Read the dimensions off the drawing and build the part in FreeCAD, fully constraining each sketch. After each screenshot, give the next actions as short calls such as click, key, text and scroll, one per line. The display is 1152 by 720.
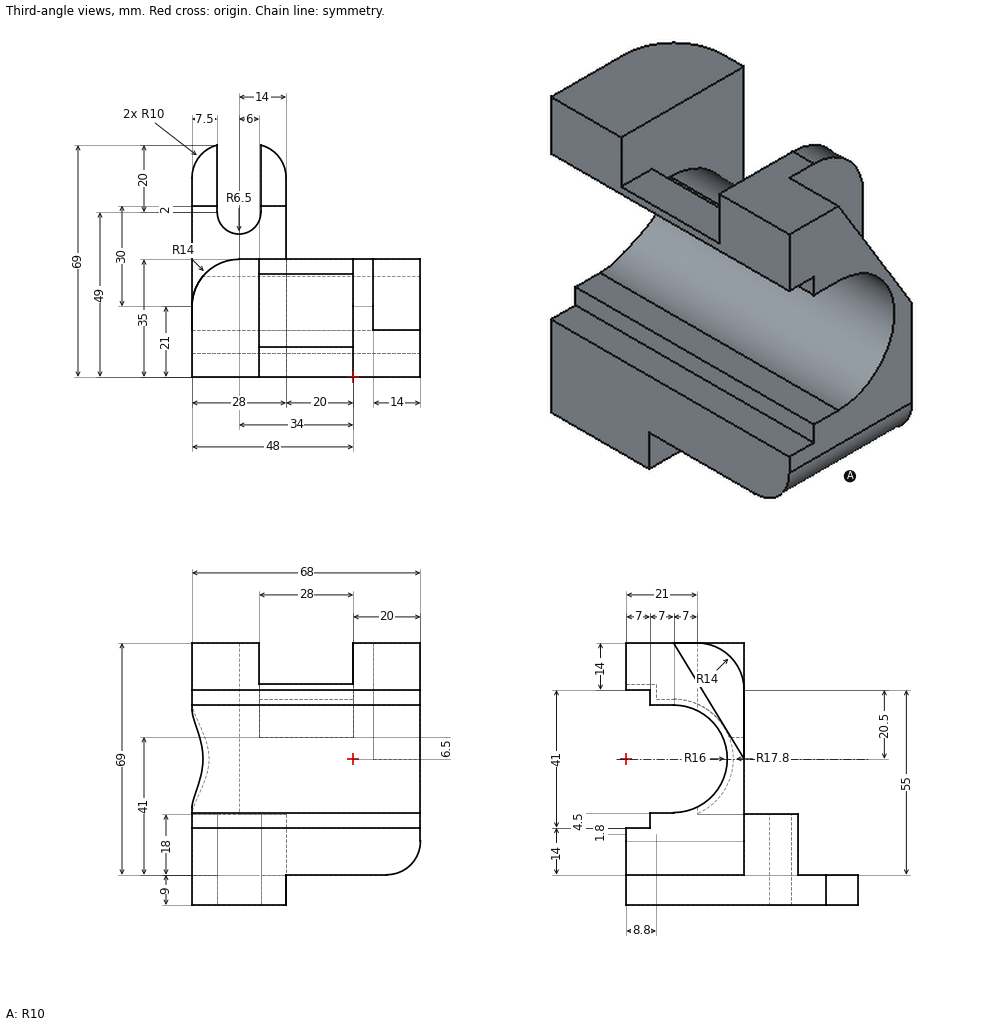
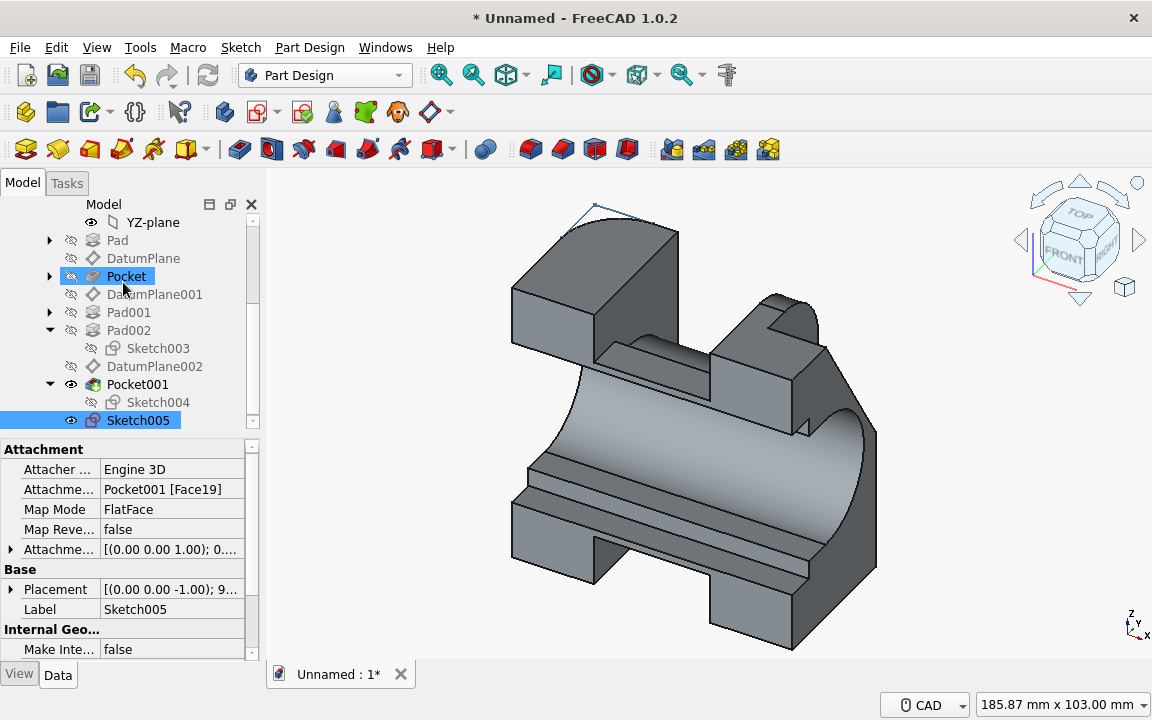
click(240, 150)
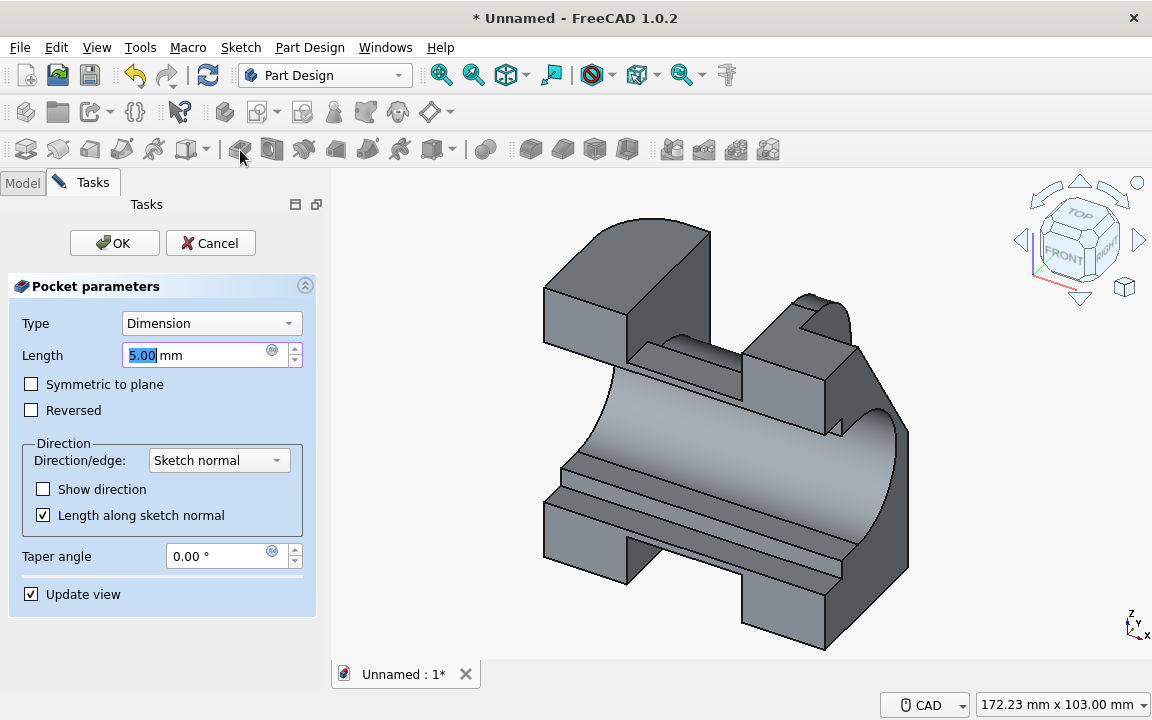
text(69)
key(Tab)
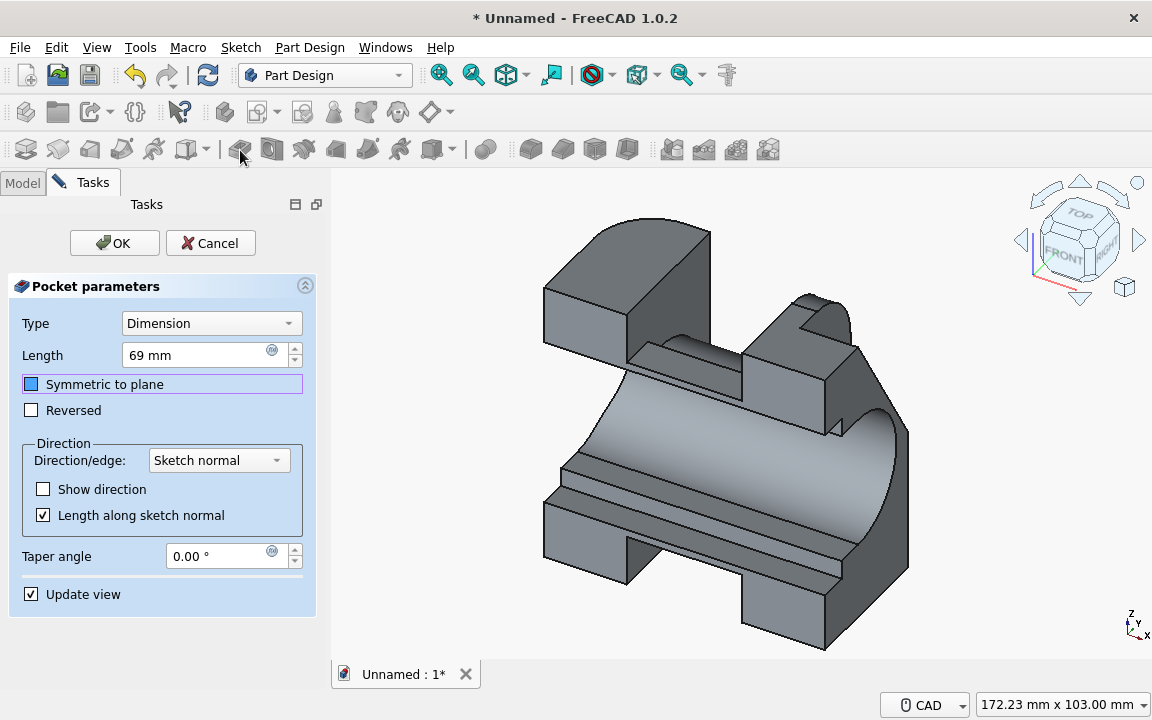
click(115, 243)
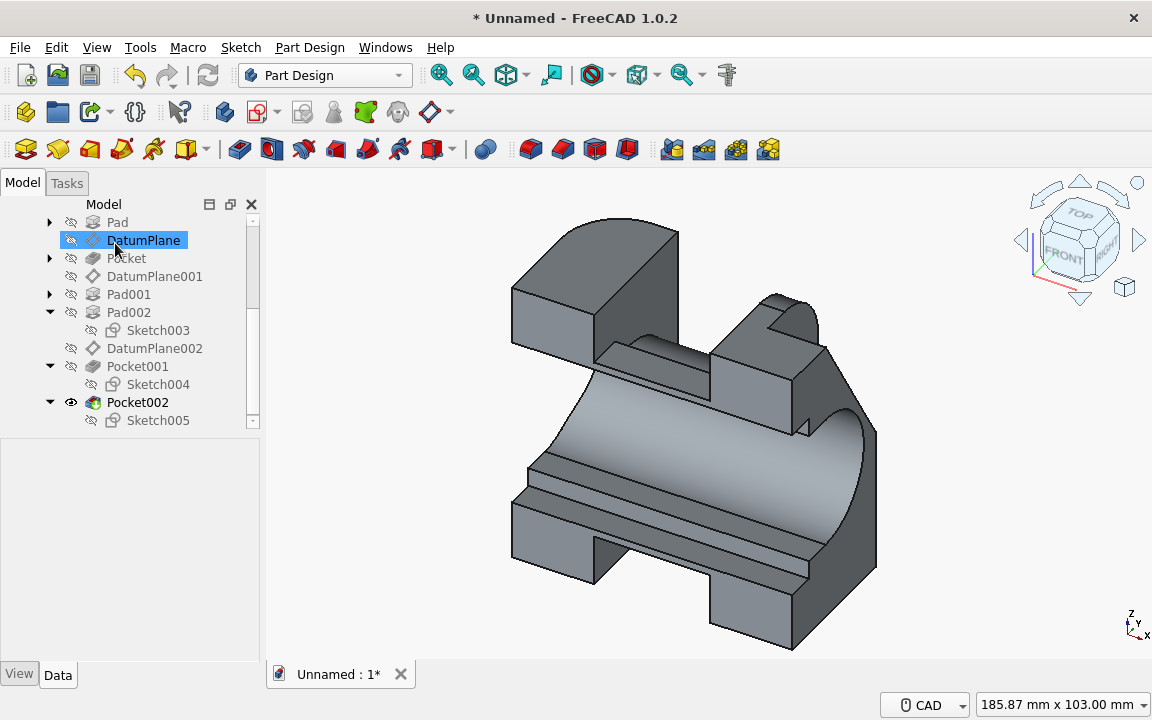
key(5)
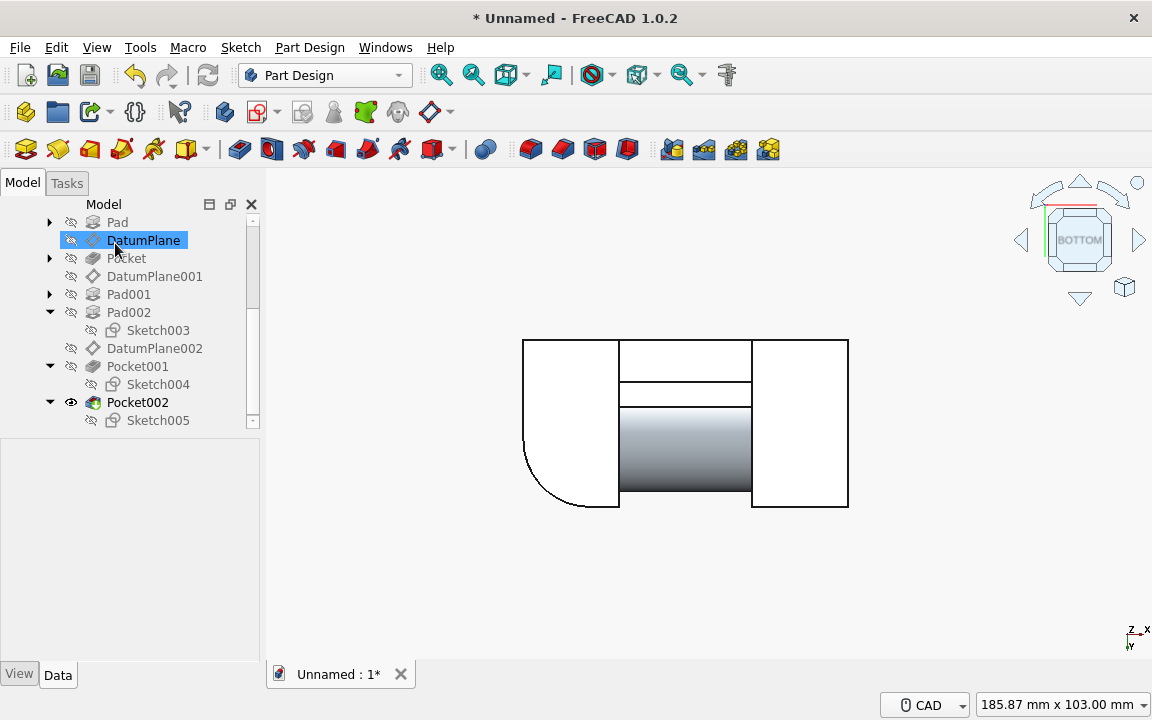
key(v)
key(f)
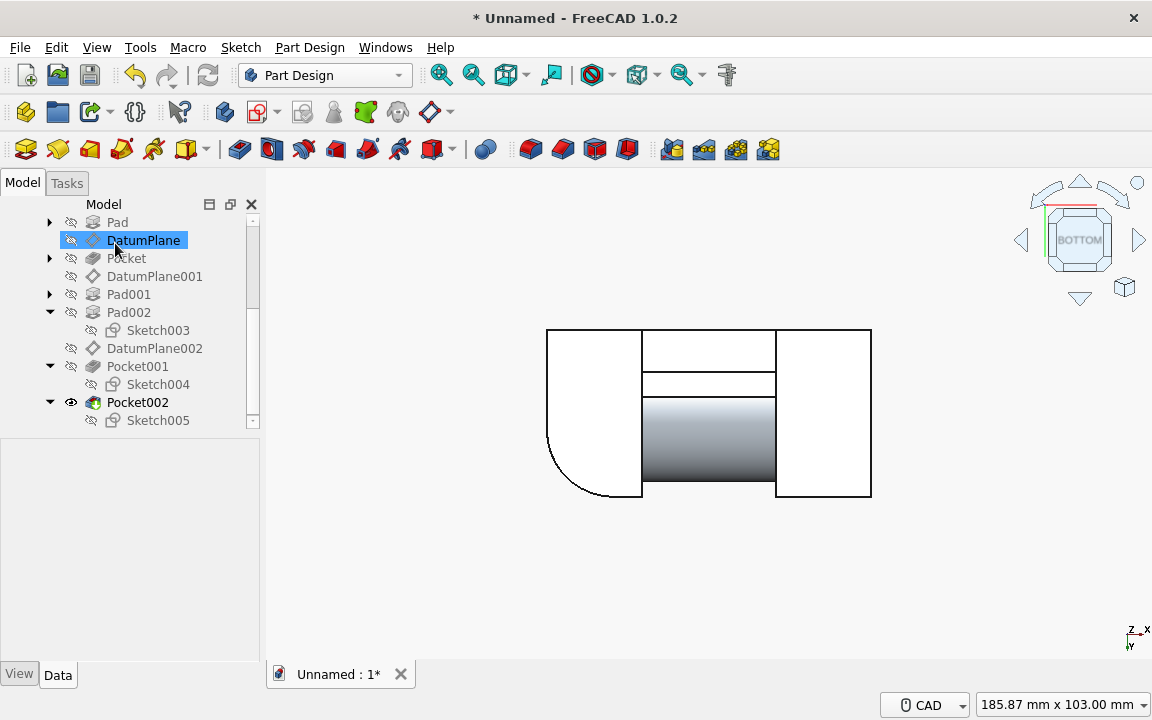
click(823, 436)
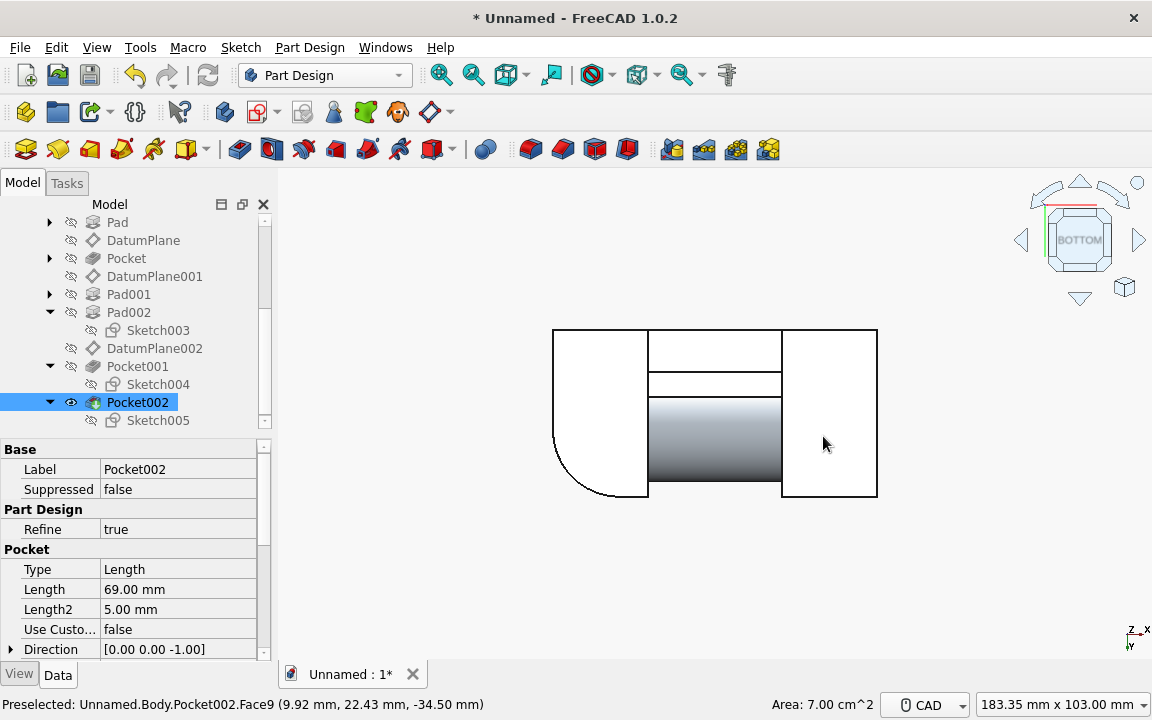
click(258, 112)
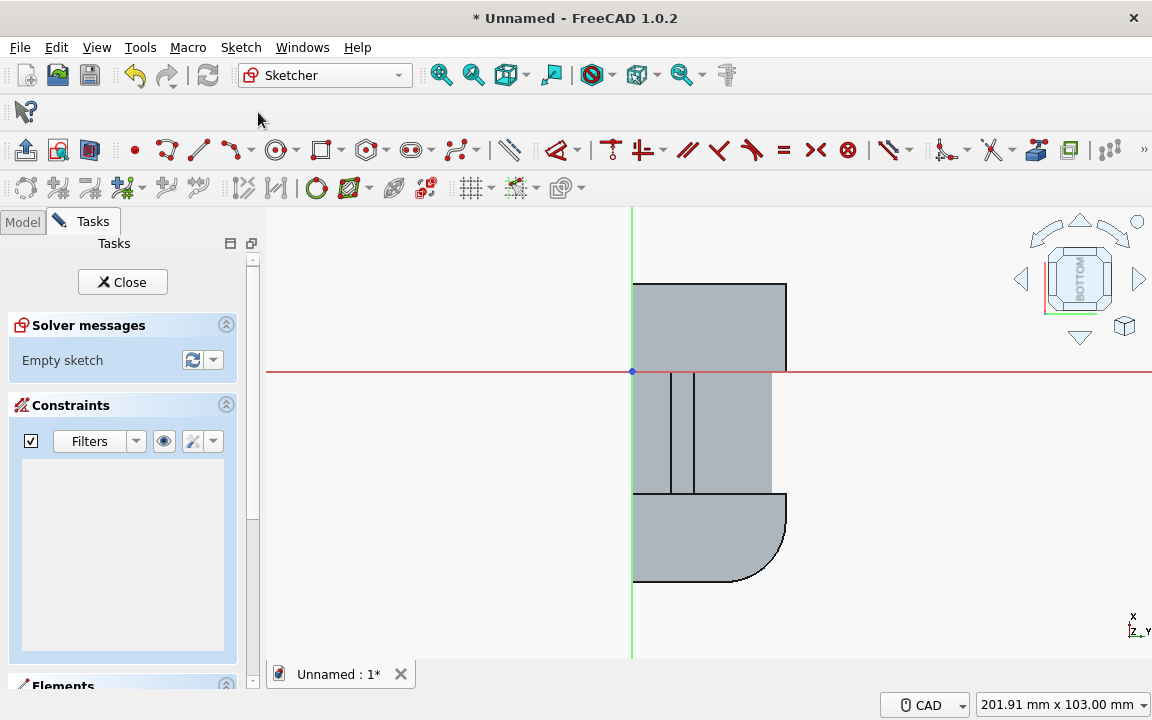
click(200, 150)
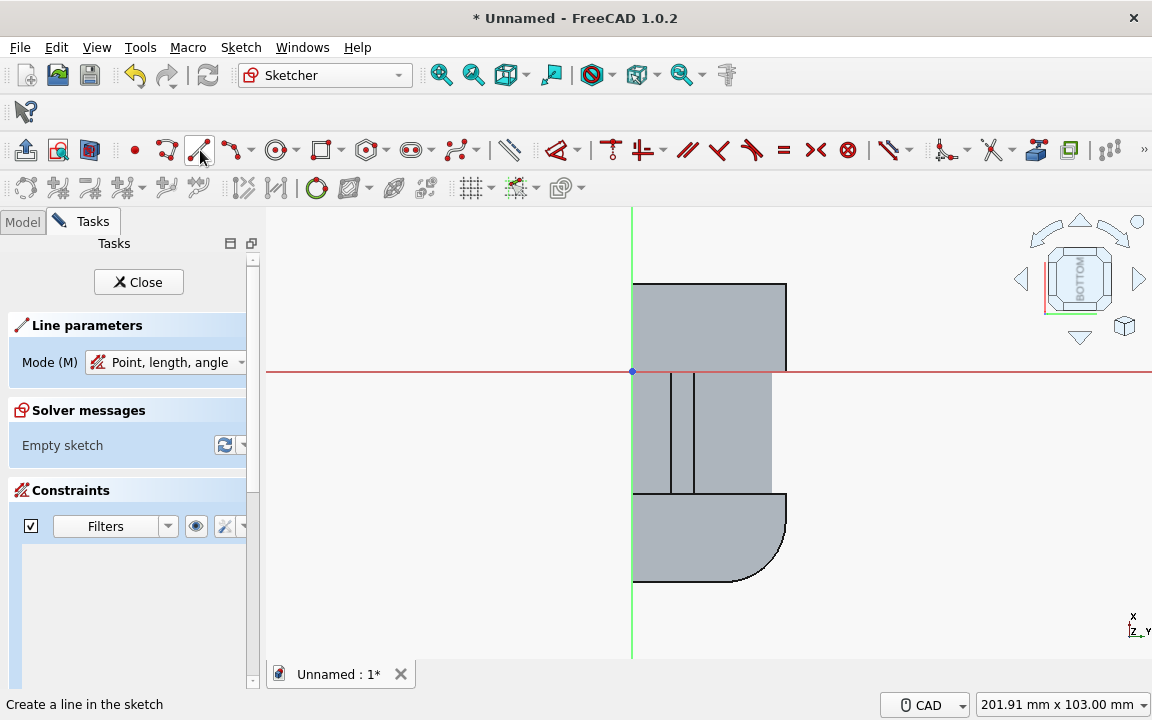
click(935, 549)
click(847, 549)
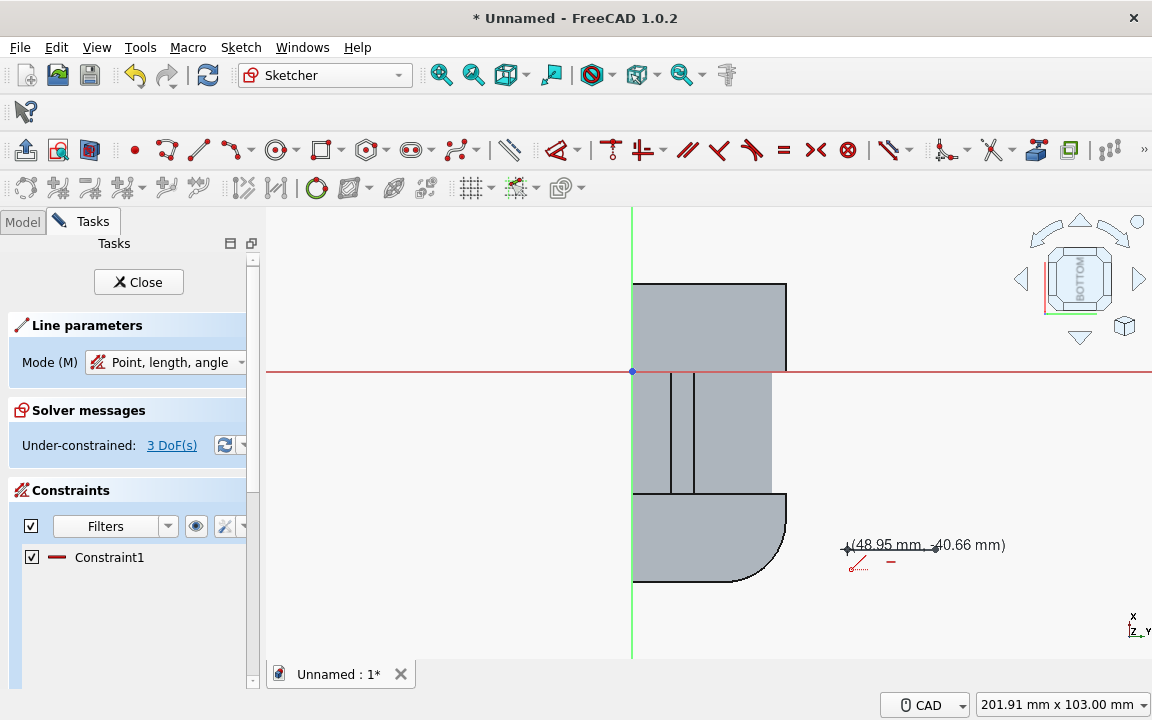
click(847, 492)
click(935, 492)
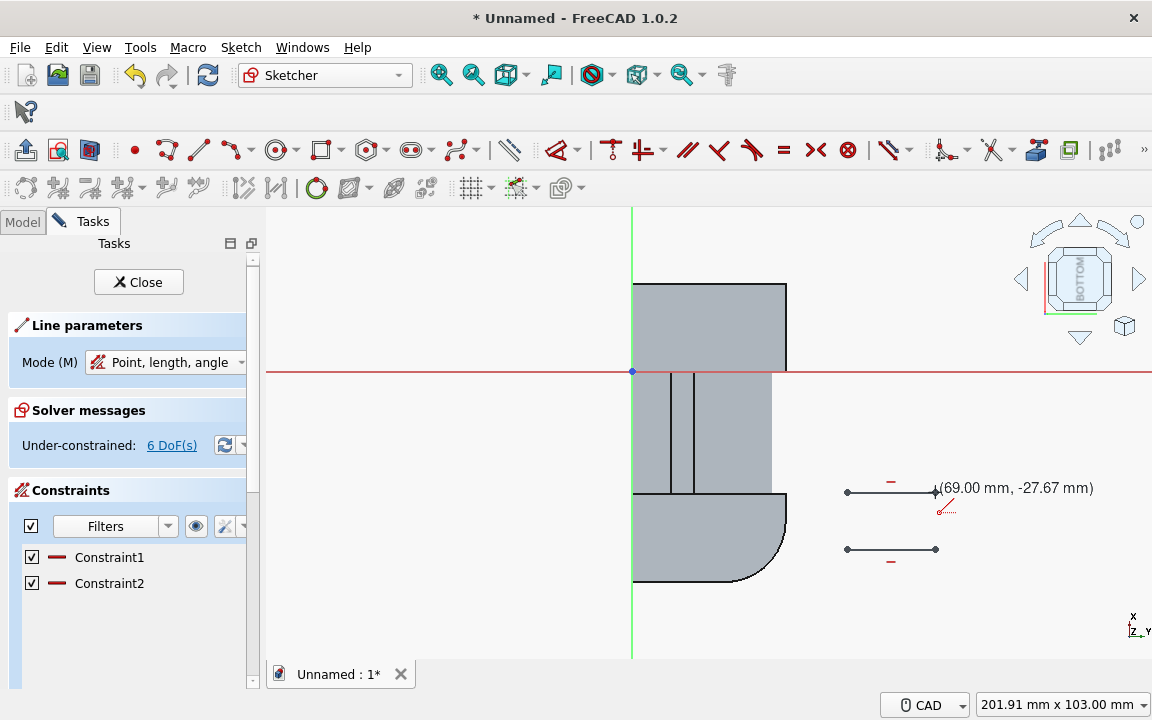
click(168, 150)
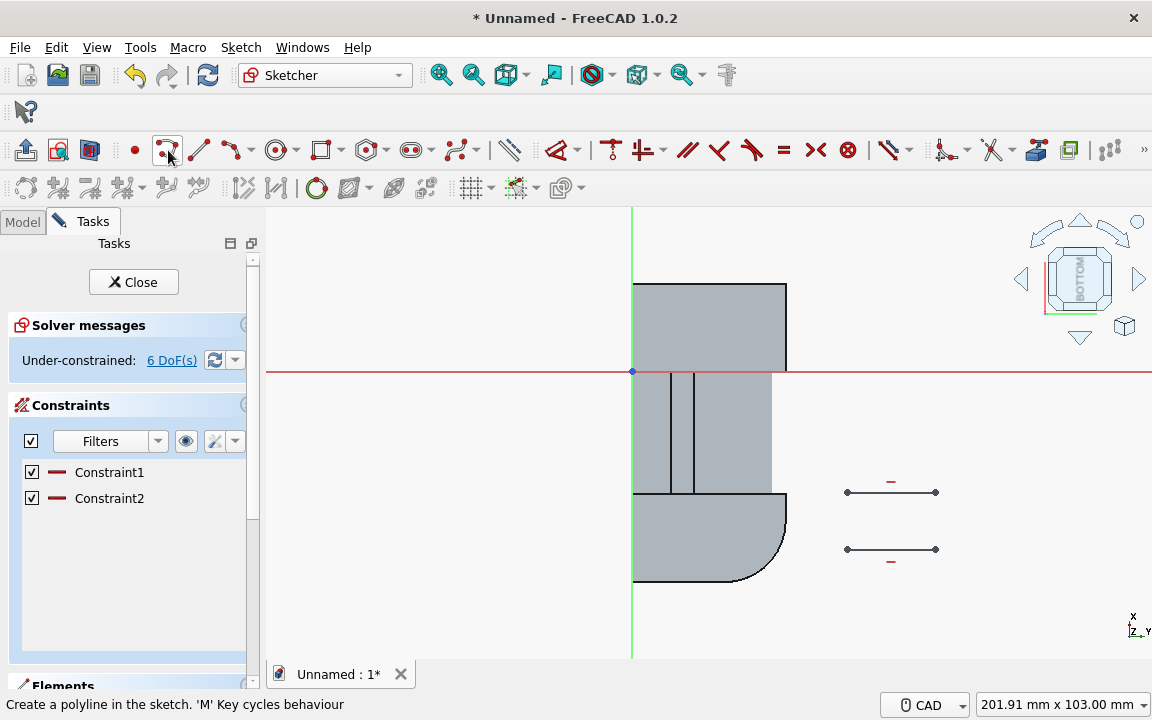
click(893, 459)
click(632, 459)
click(641, 582)
click(893, 582)
right_click(893, 582)